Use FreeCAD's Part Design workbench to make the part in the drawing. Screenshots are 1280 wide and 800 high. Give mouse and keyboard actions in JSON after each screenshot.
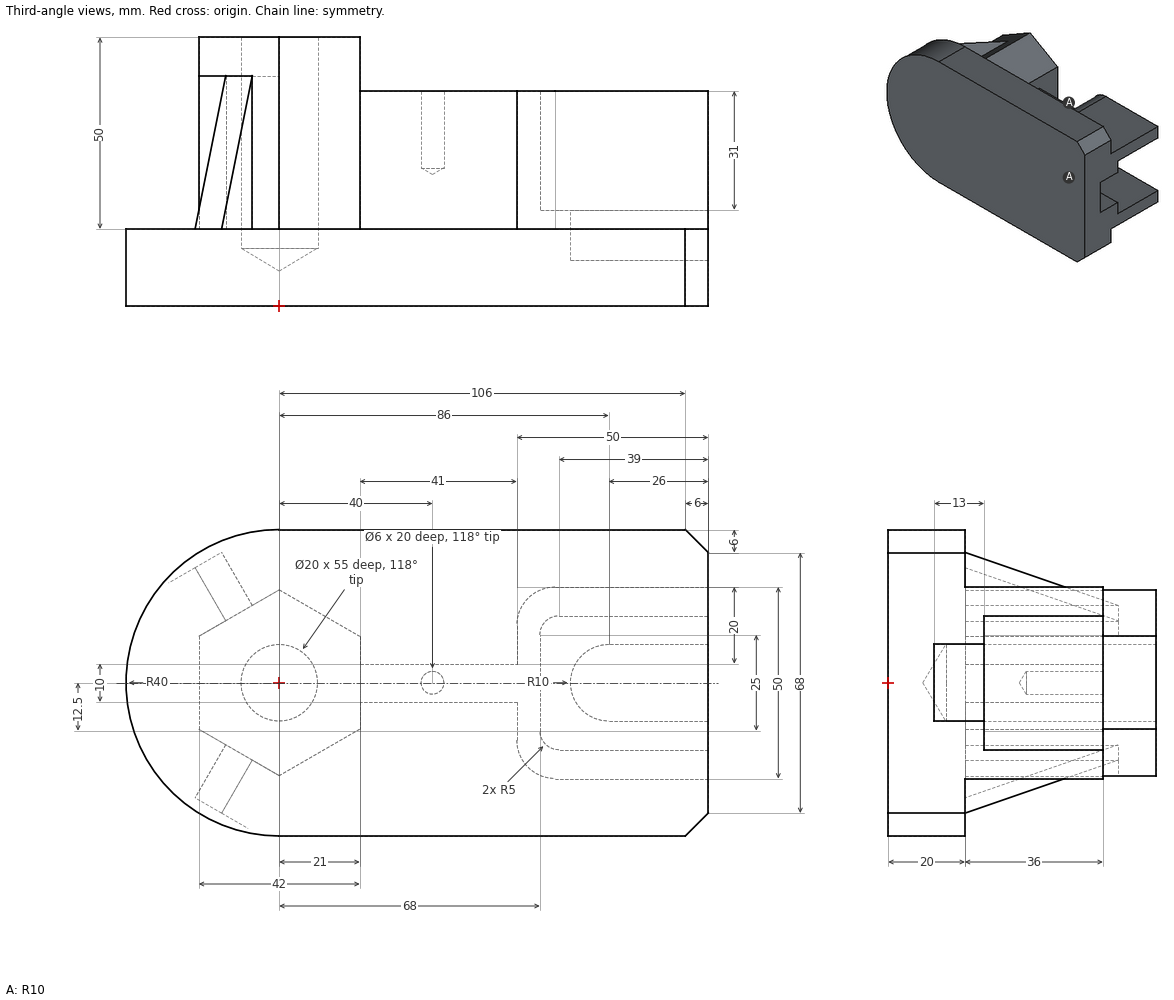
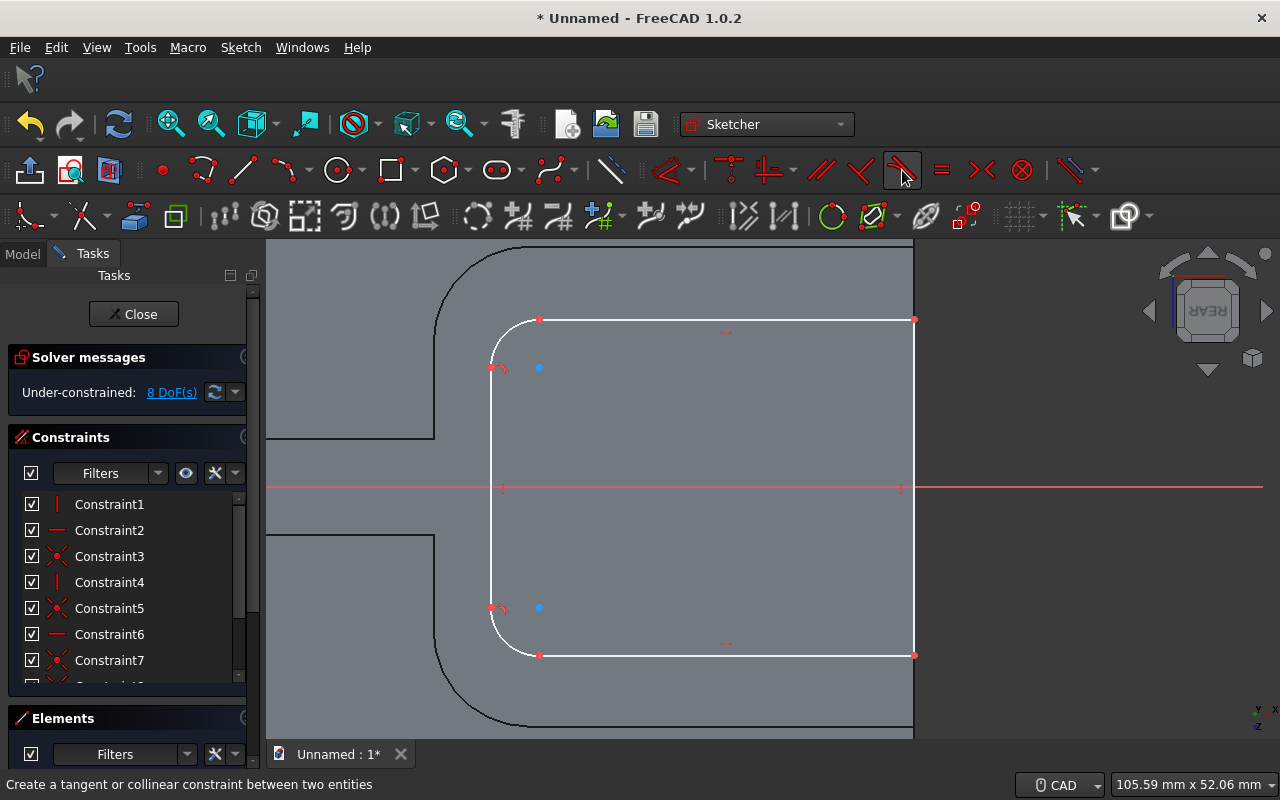
{"action": "left_click", "coordinate": [652, 656]}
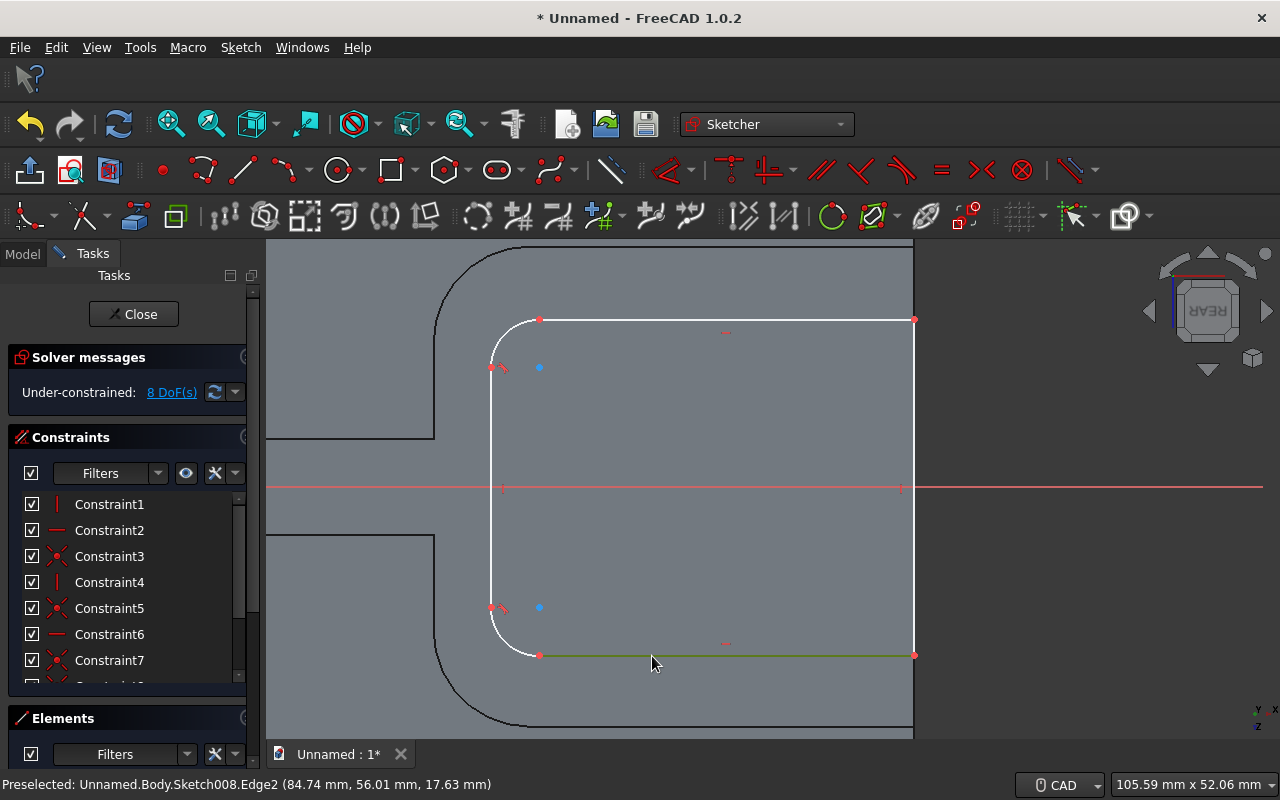
{"action": "left_click", "coordinate": [496, 630]}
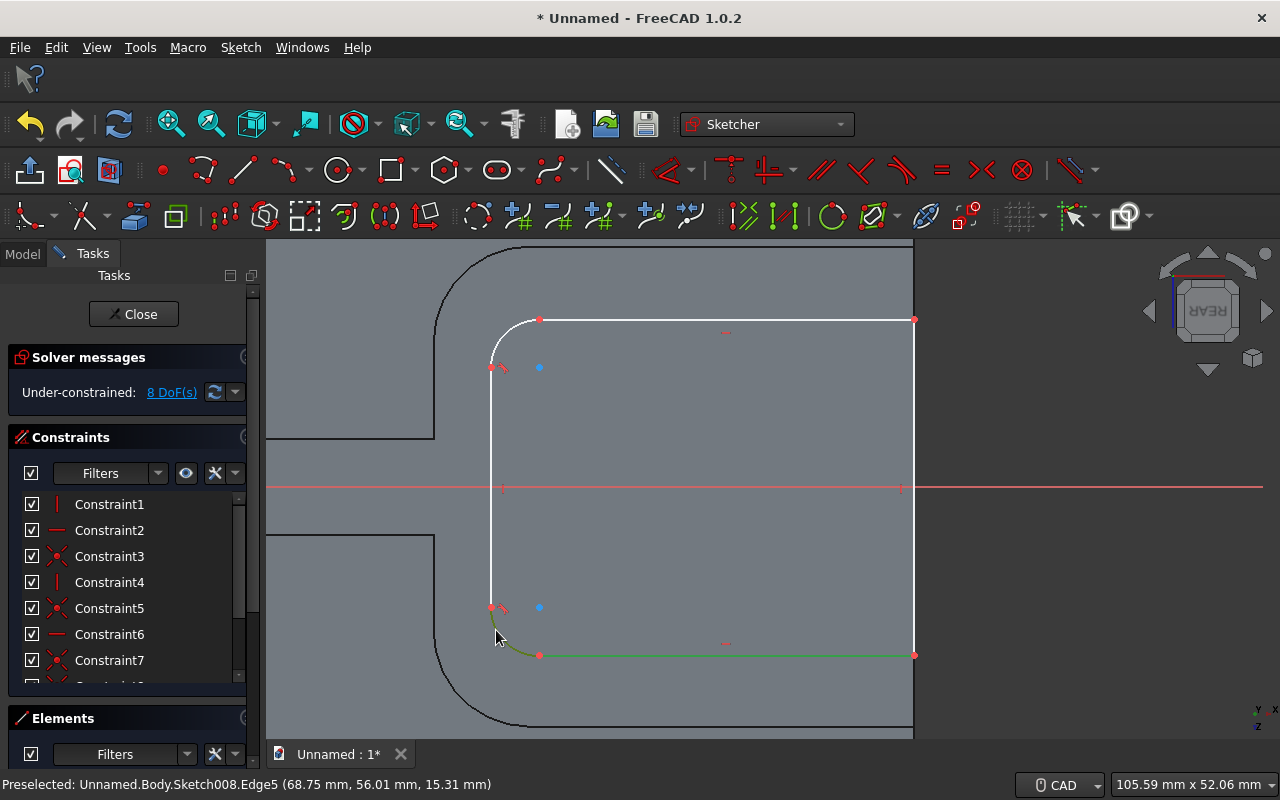
{"action": "left_click", "coordinate": [902, 170]}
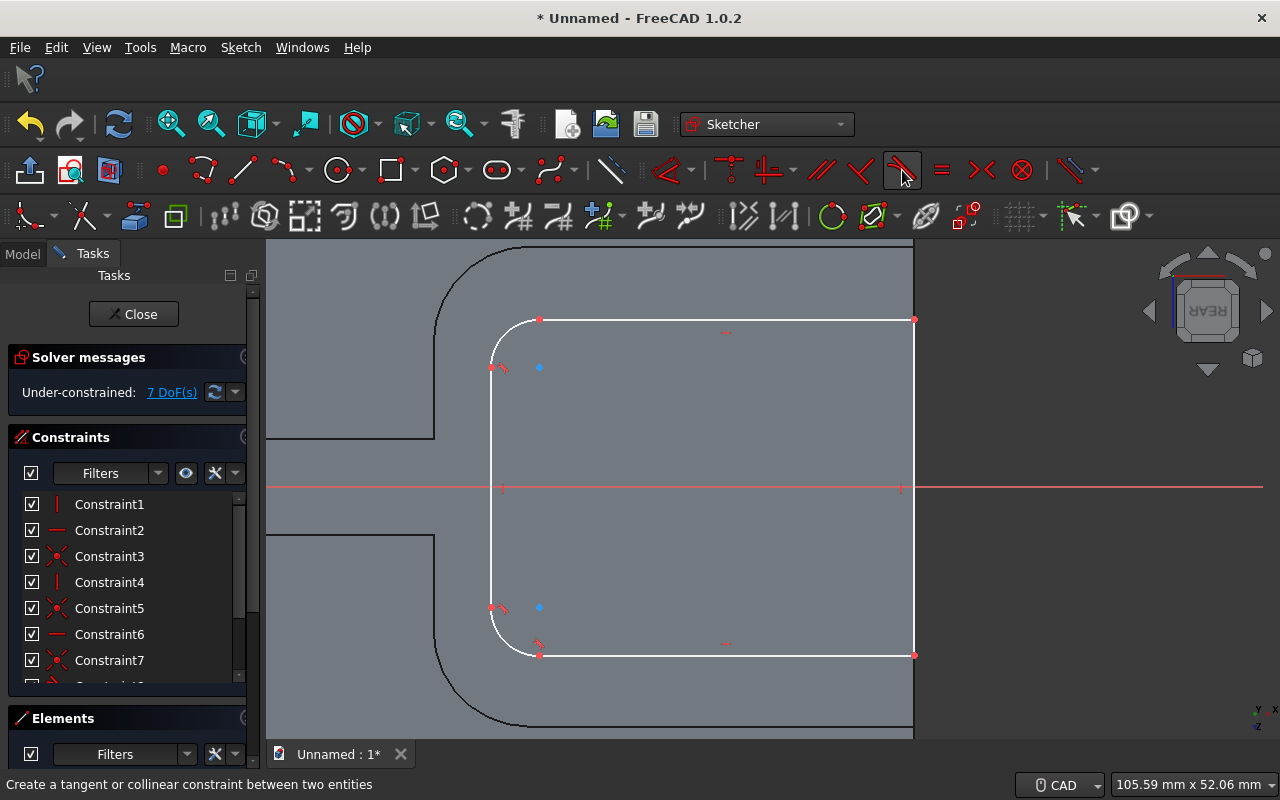
{"action": "left_click", "coordinate": [801, 320]}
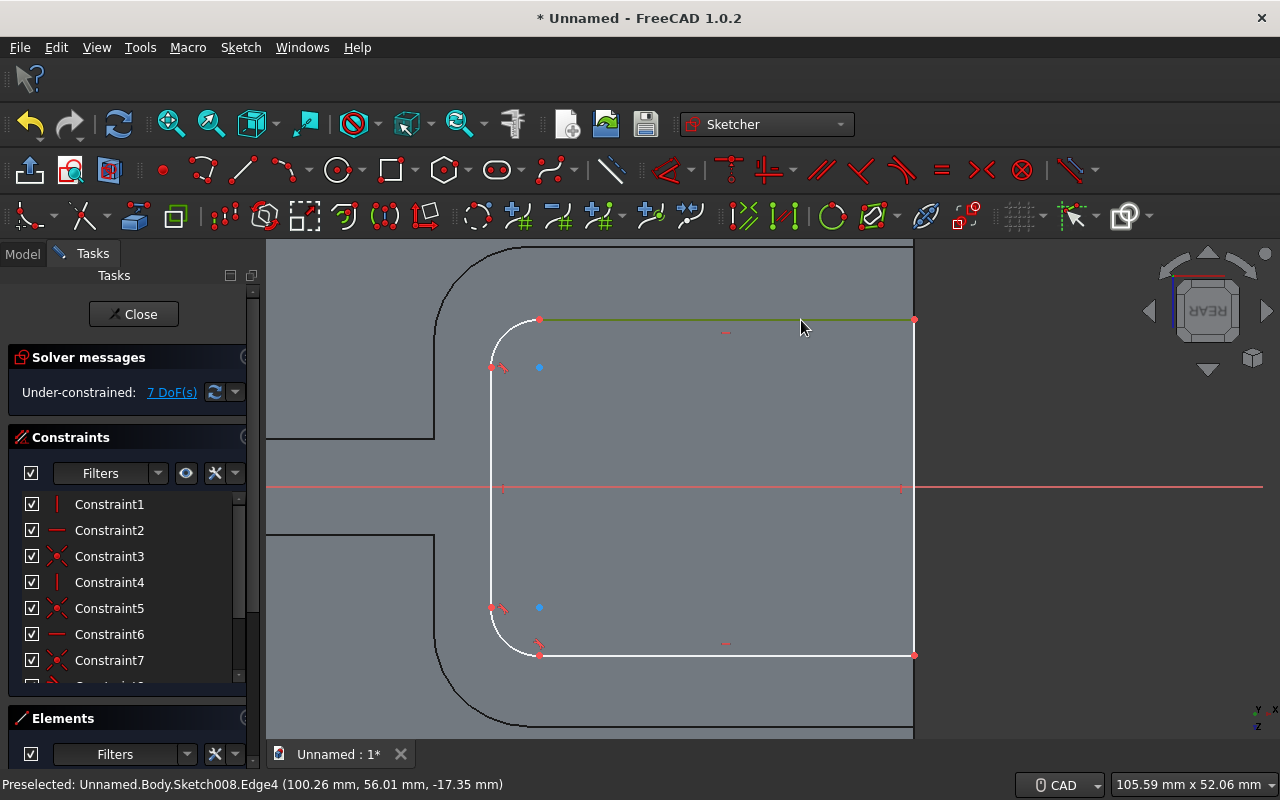
{"action": "left_click", "coordinate": [517, 325]}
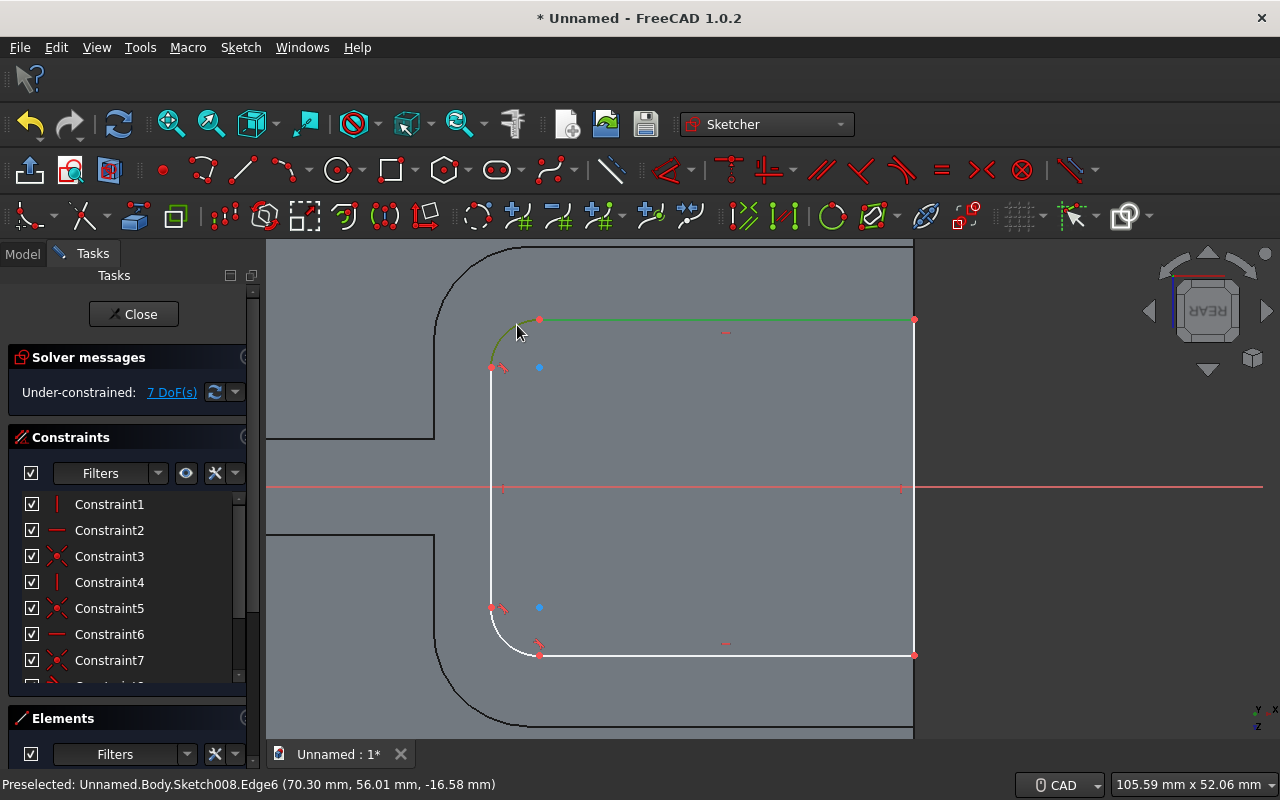
{"action": "left_click", "coordinate": [902, 170]}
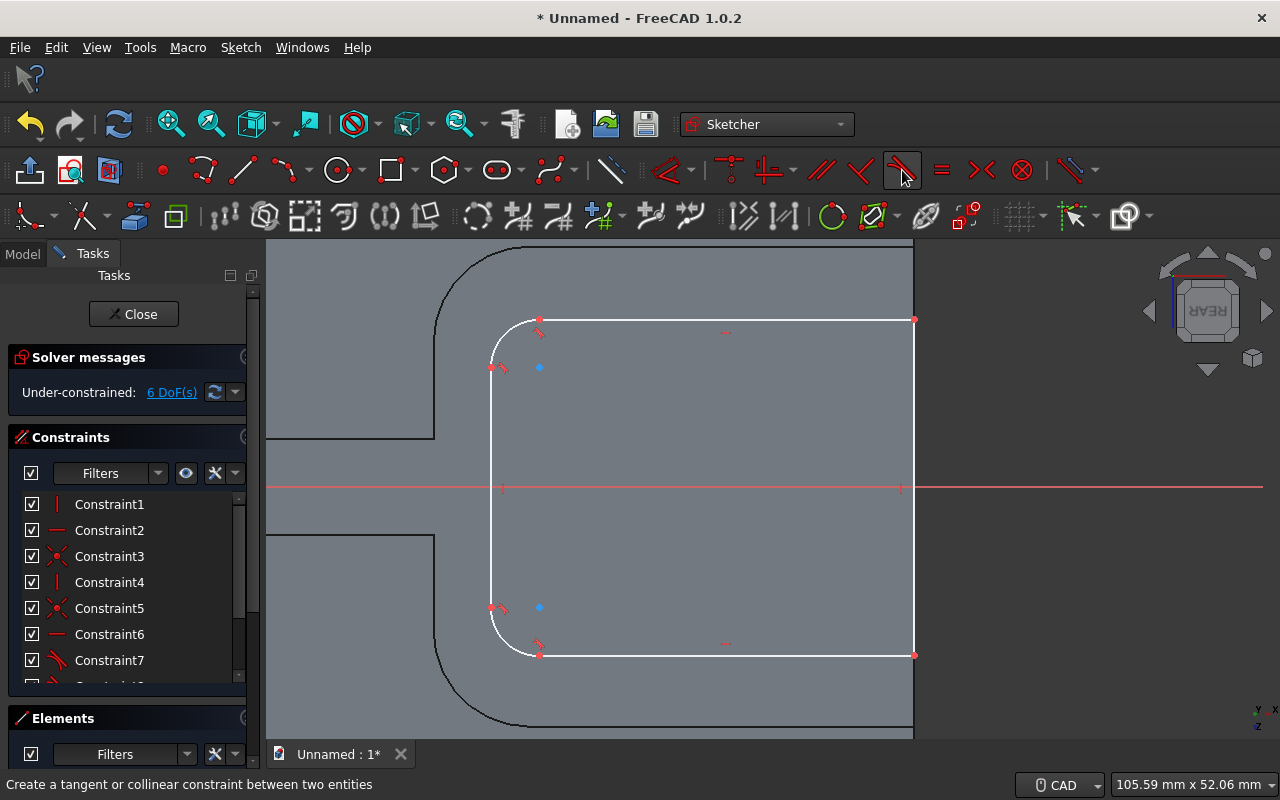
{"action": "left_click", "coordinate": [496, 630]}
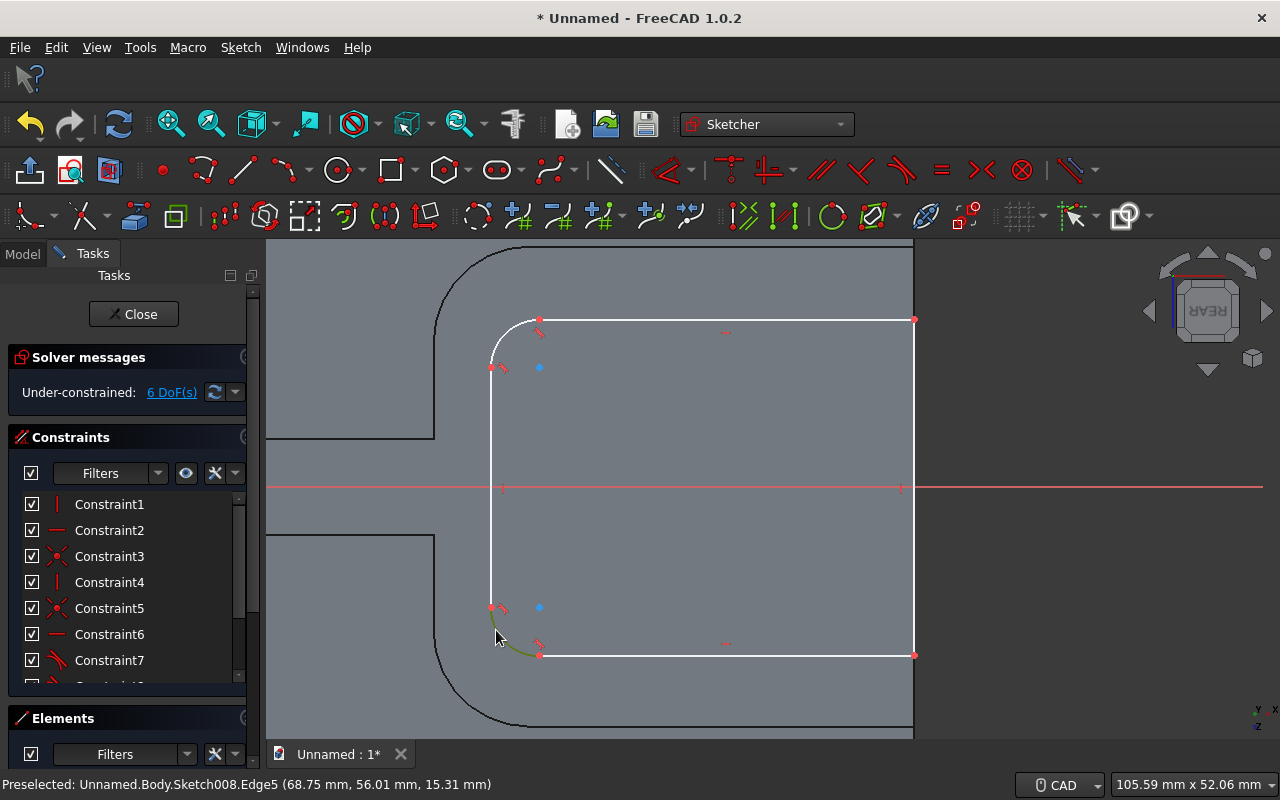
{"action": "left_click", "coordinate": [517, 325]}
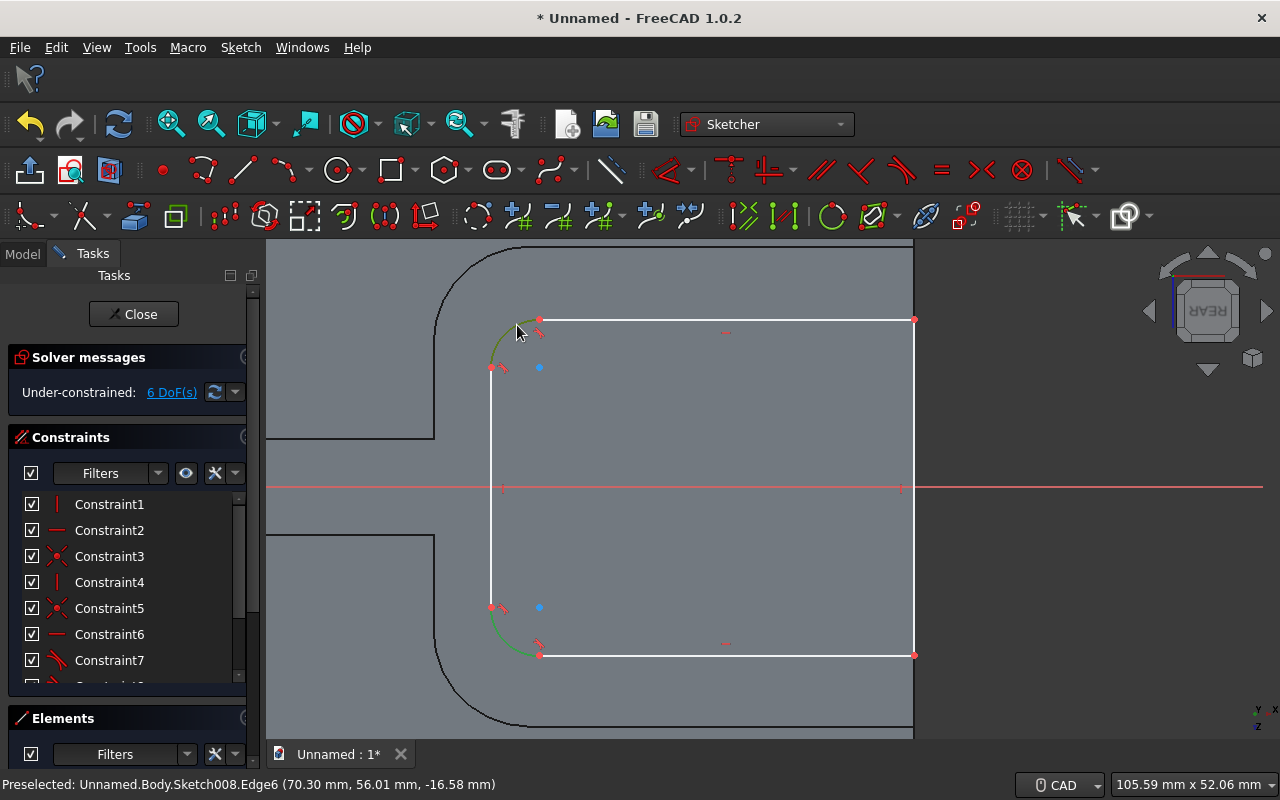
{"action": "left_click", "coordinate": [942, 170]}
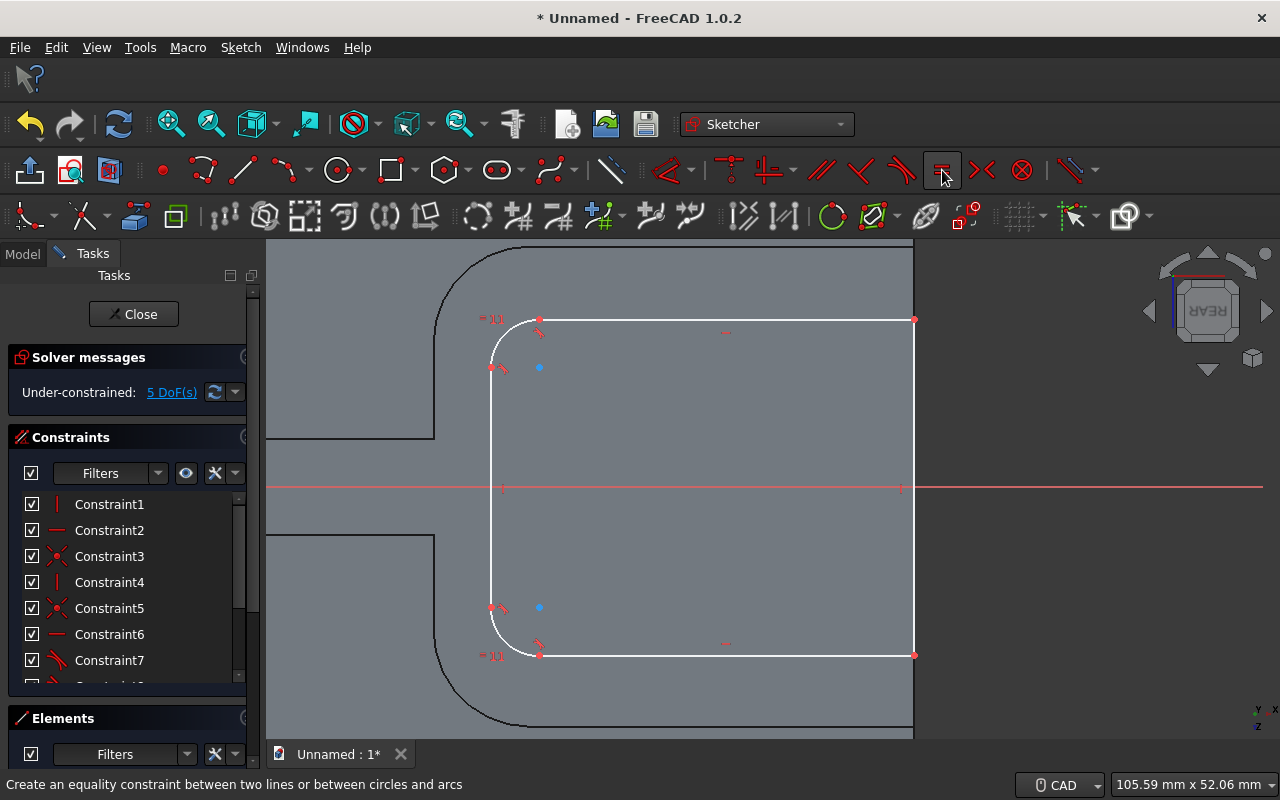
{"action": "left_click", "coordinate": [666, 170]}